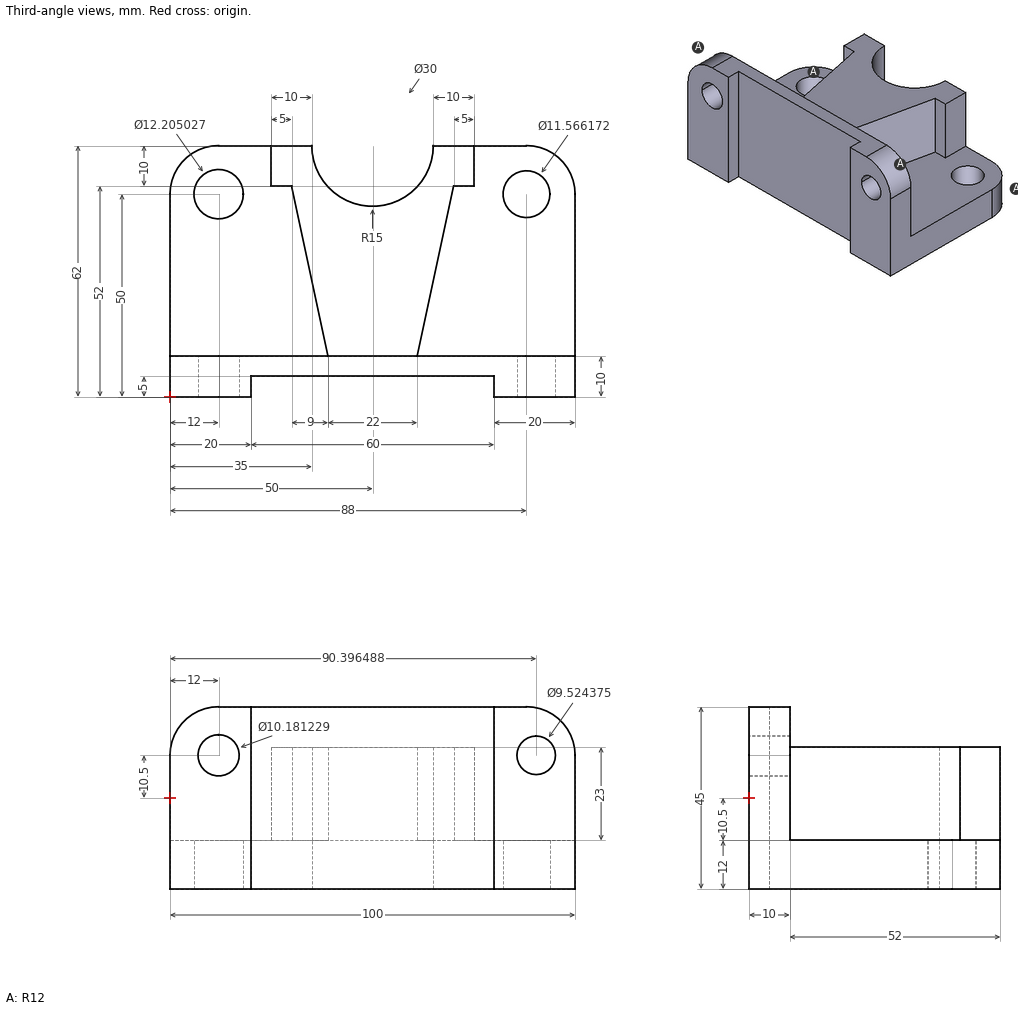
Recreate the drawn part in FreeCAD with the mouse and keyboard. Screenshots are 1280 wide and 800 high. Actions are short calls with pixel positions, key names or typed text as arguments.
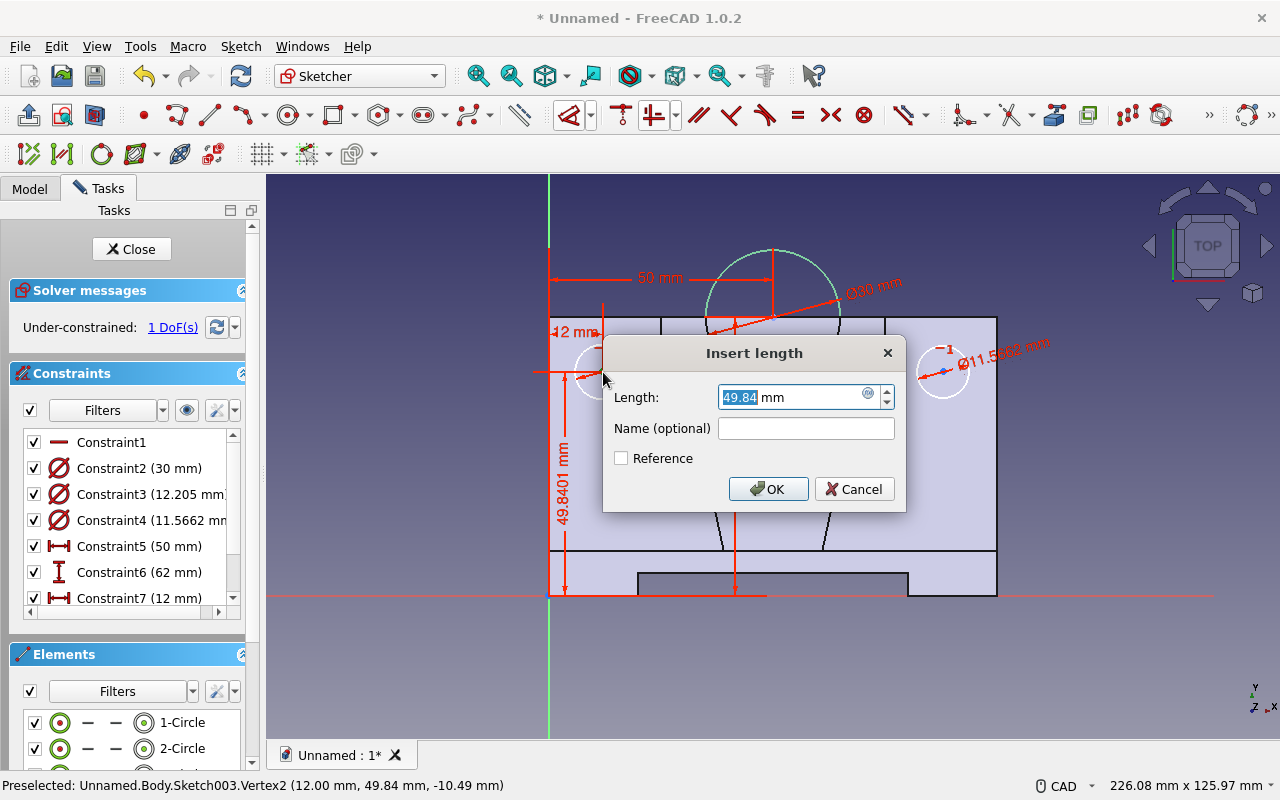
text(50)
key(Return)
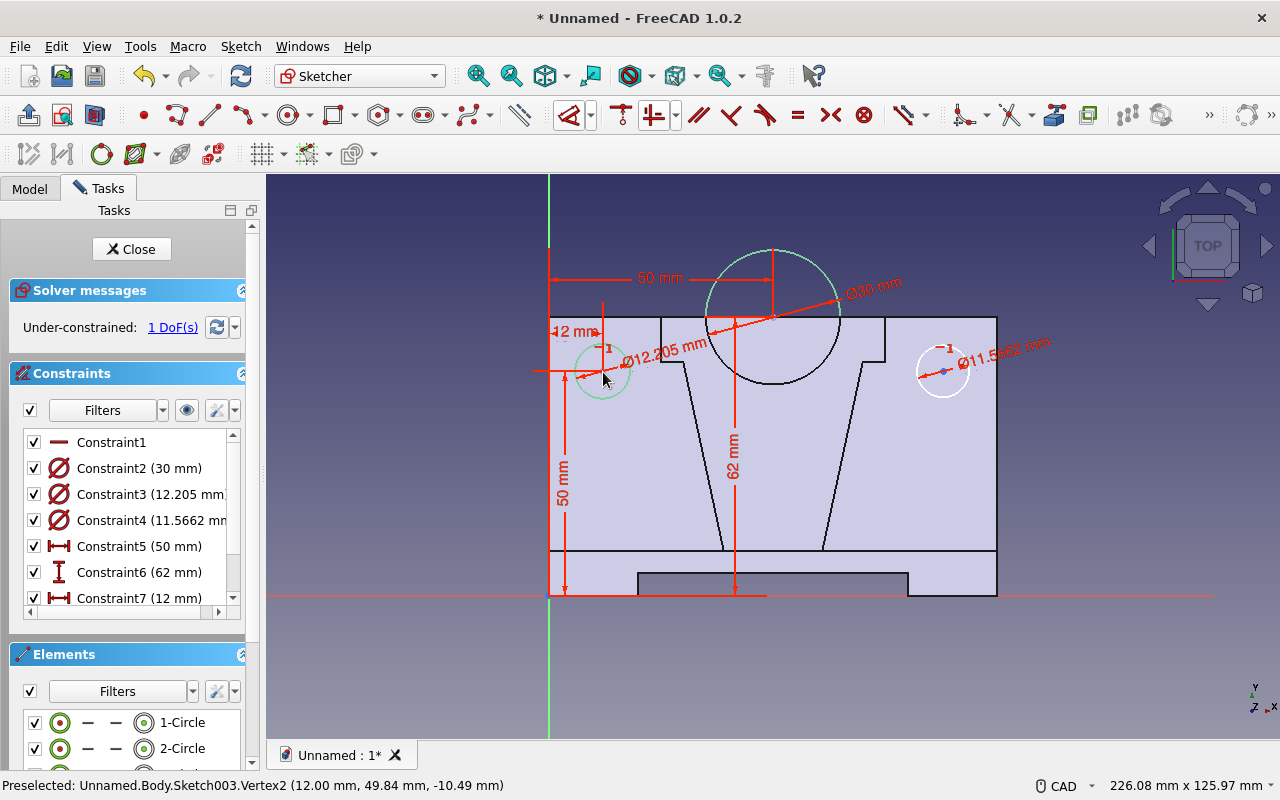
click(943, 371)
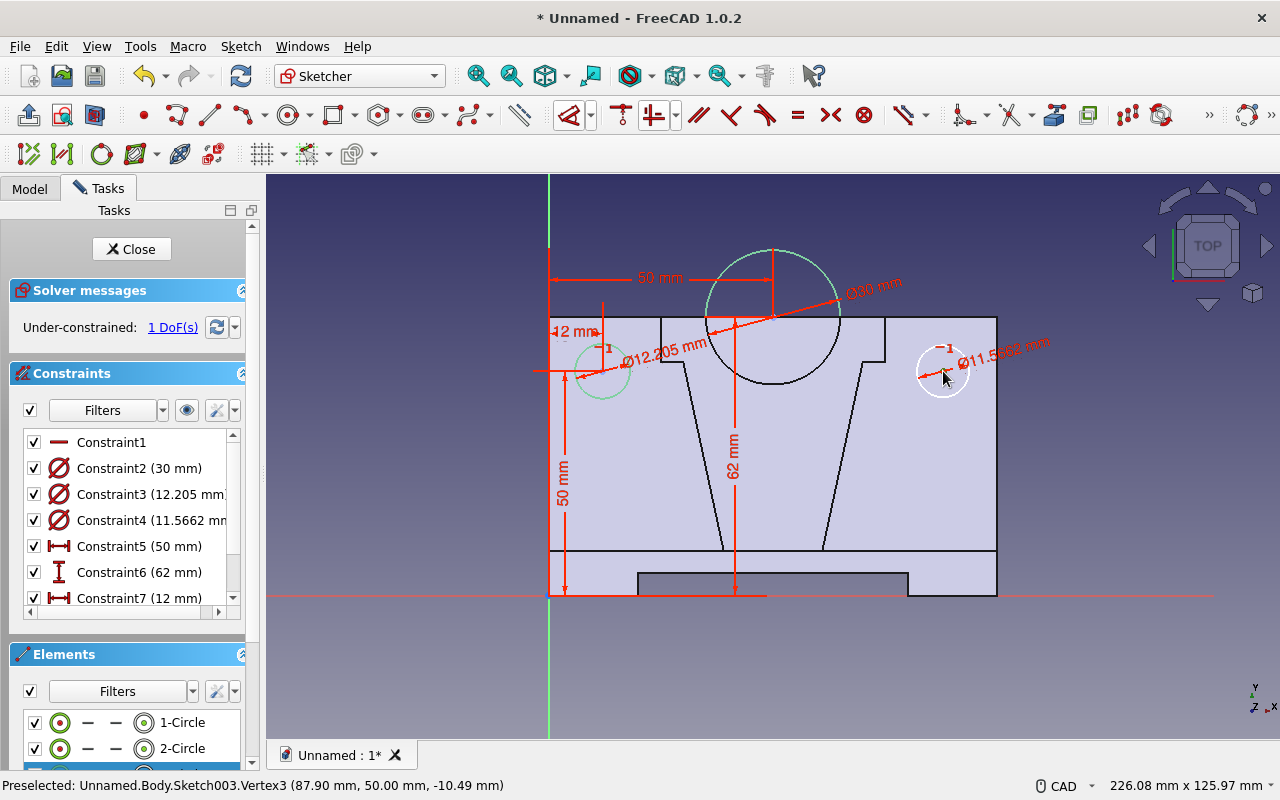
click(590, 116)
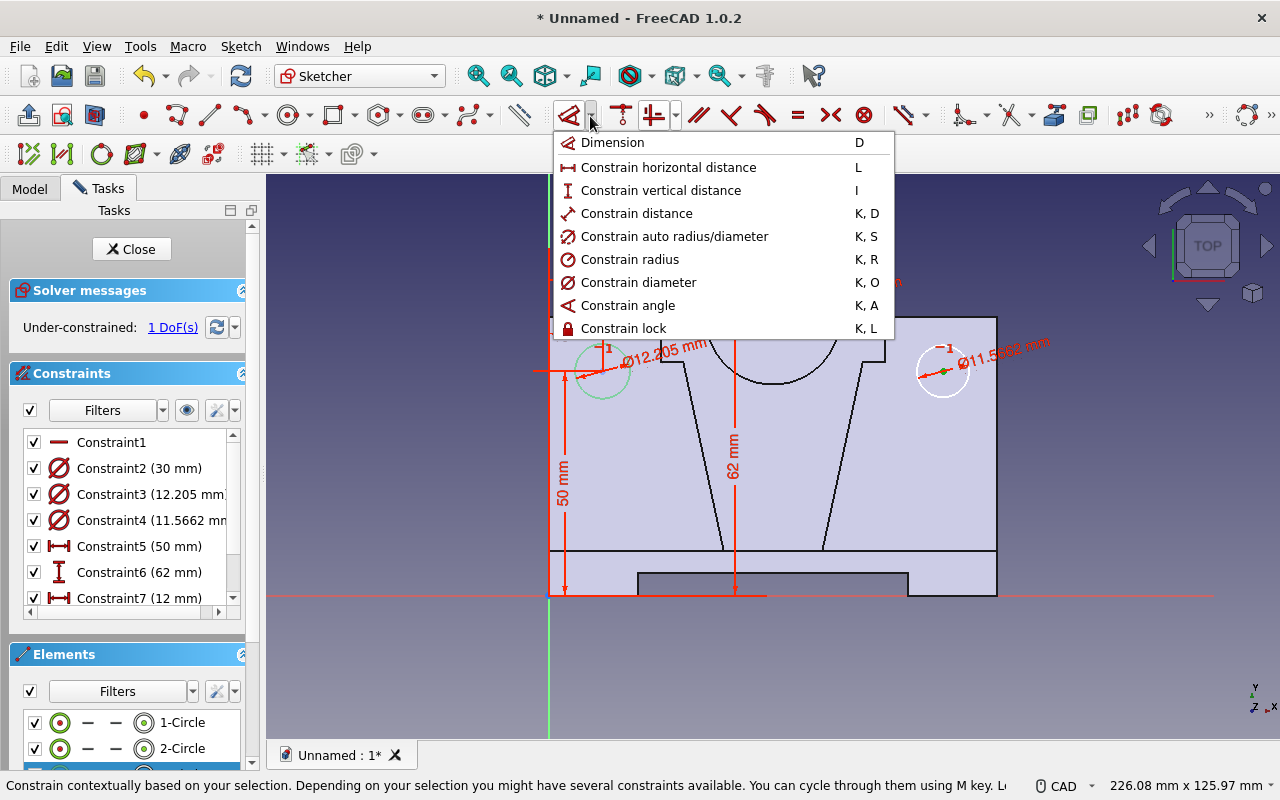
click(724, 168)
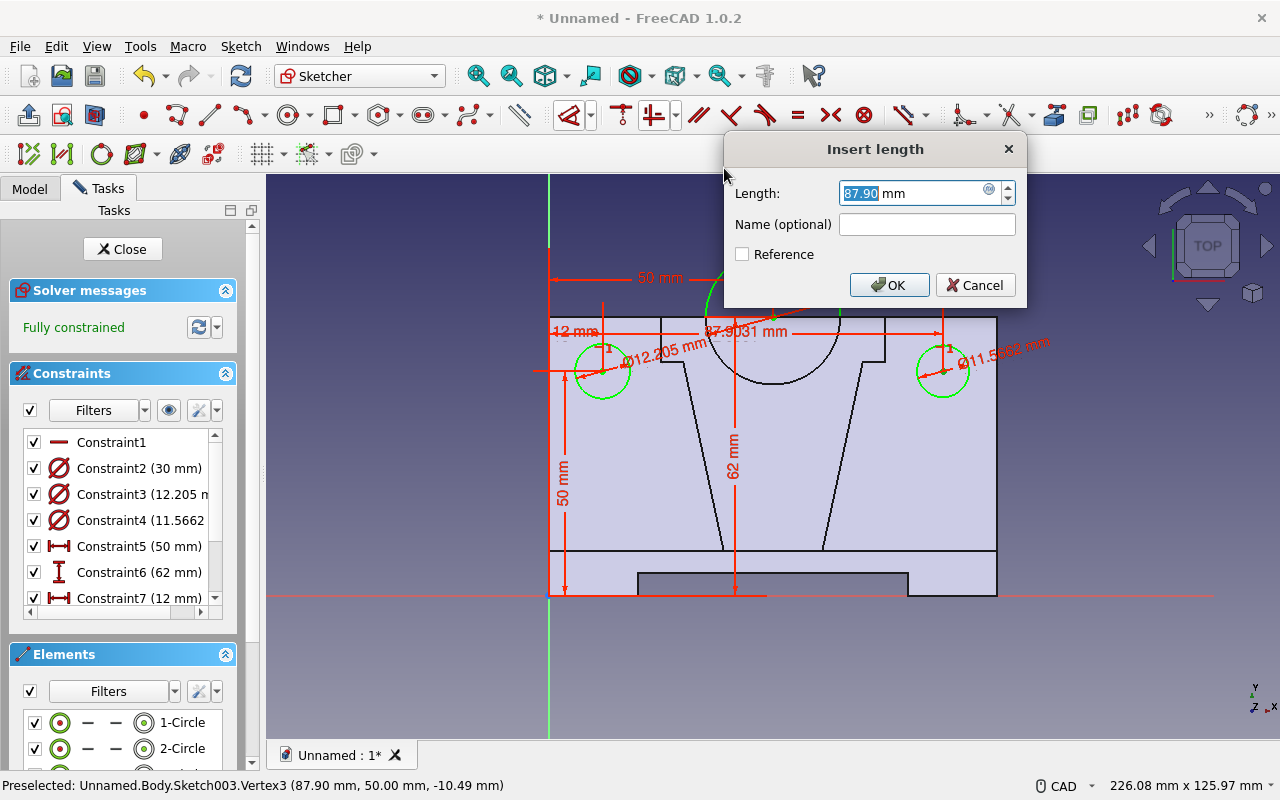
text(88)
key(Return)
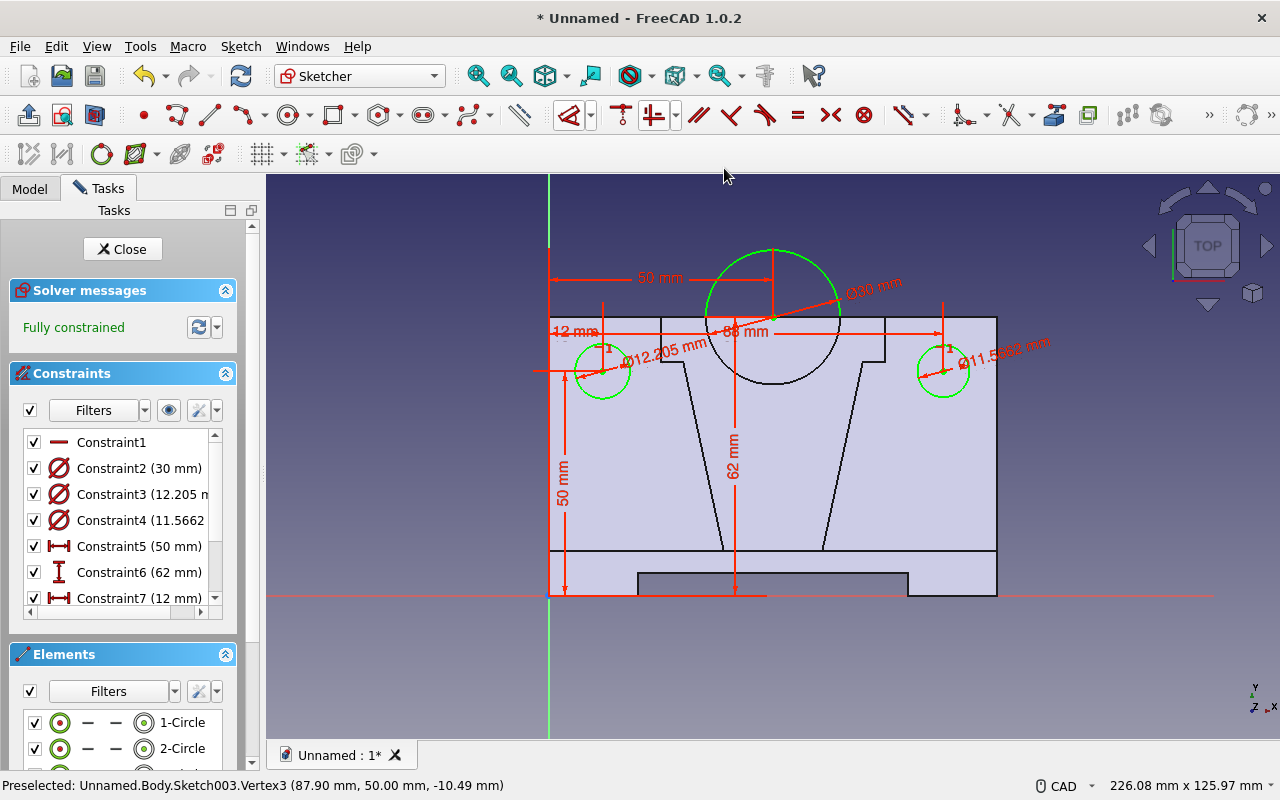
click(123, 249)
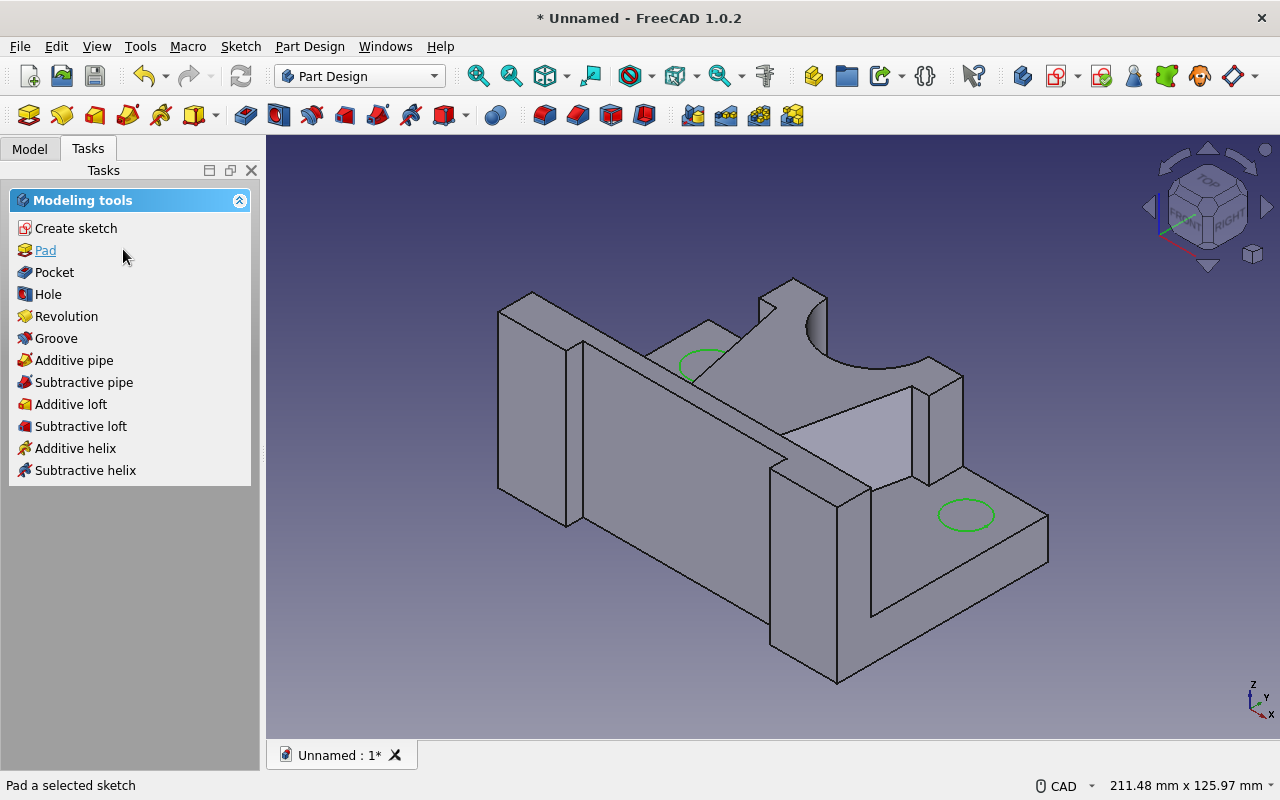
click(246, 116)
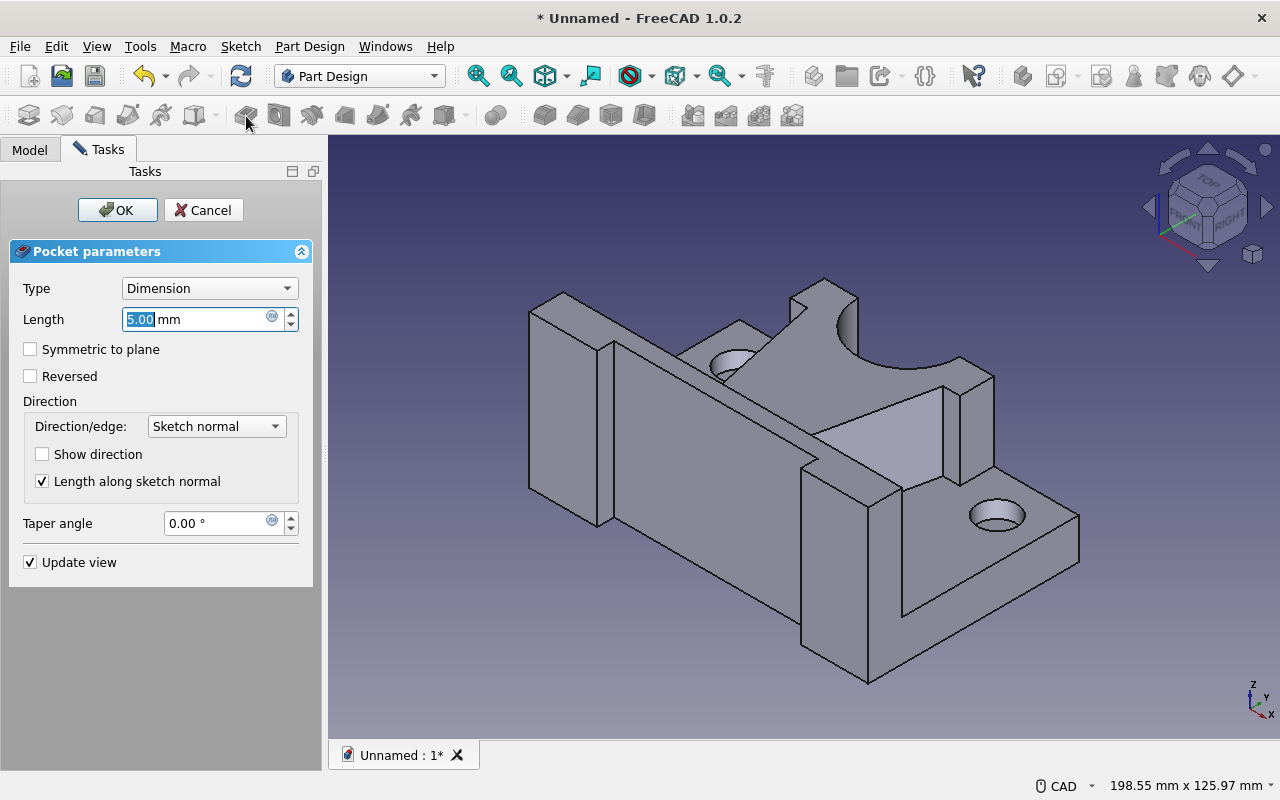
click(210, 288)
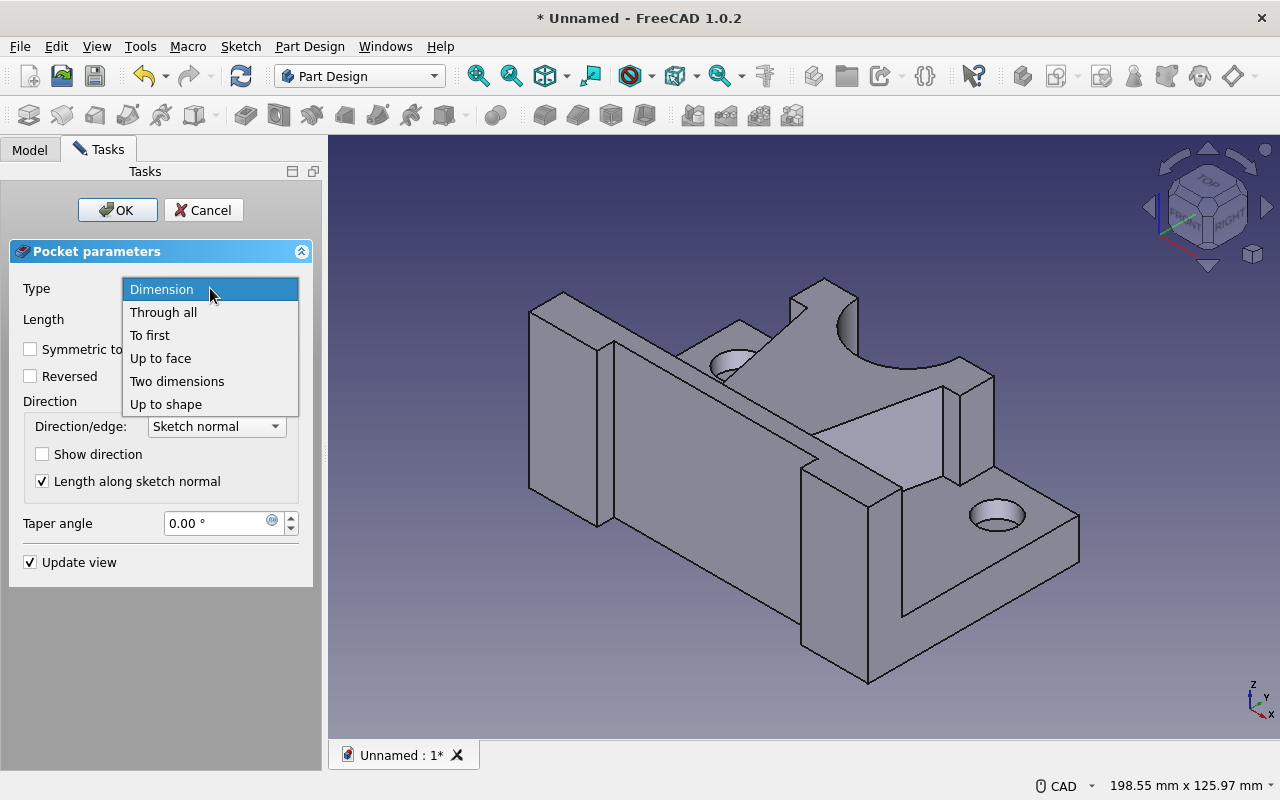
click(208, 312)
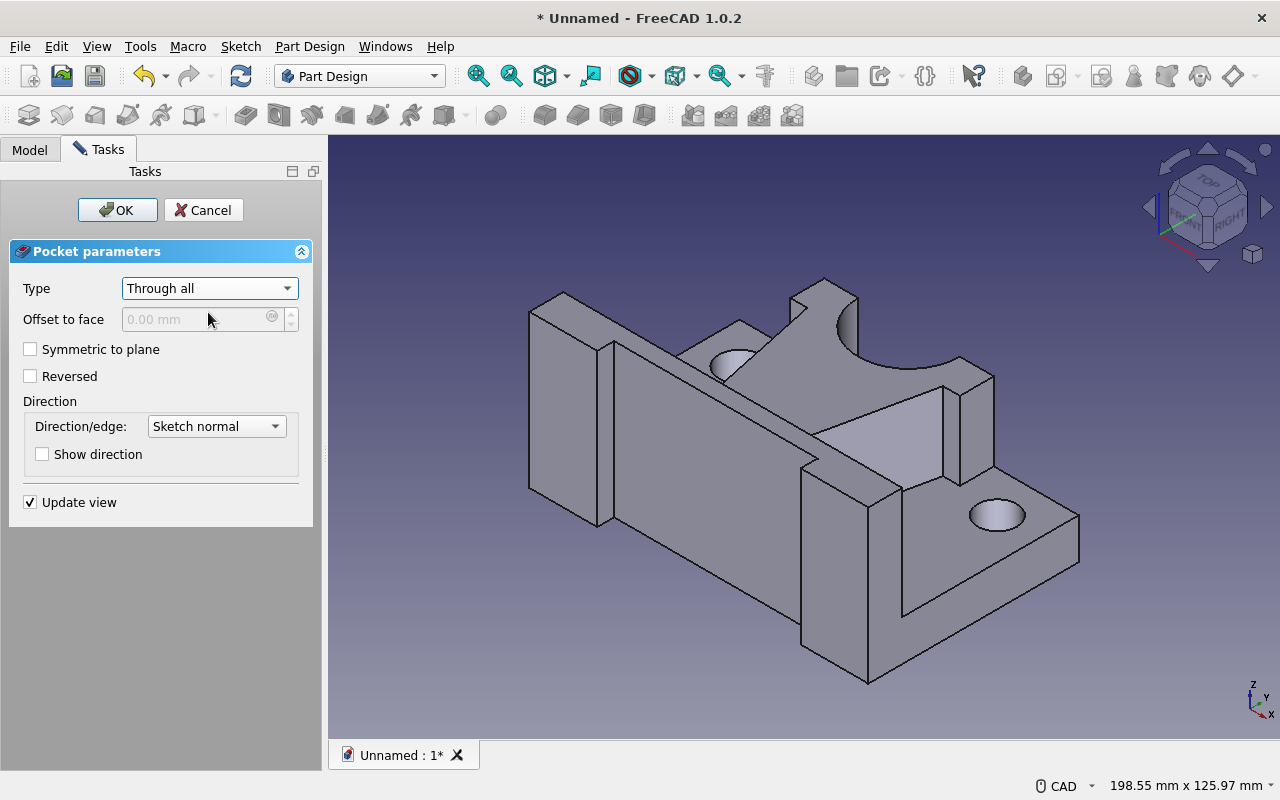
click(118, 210)